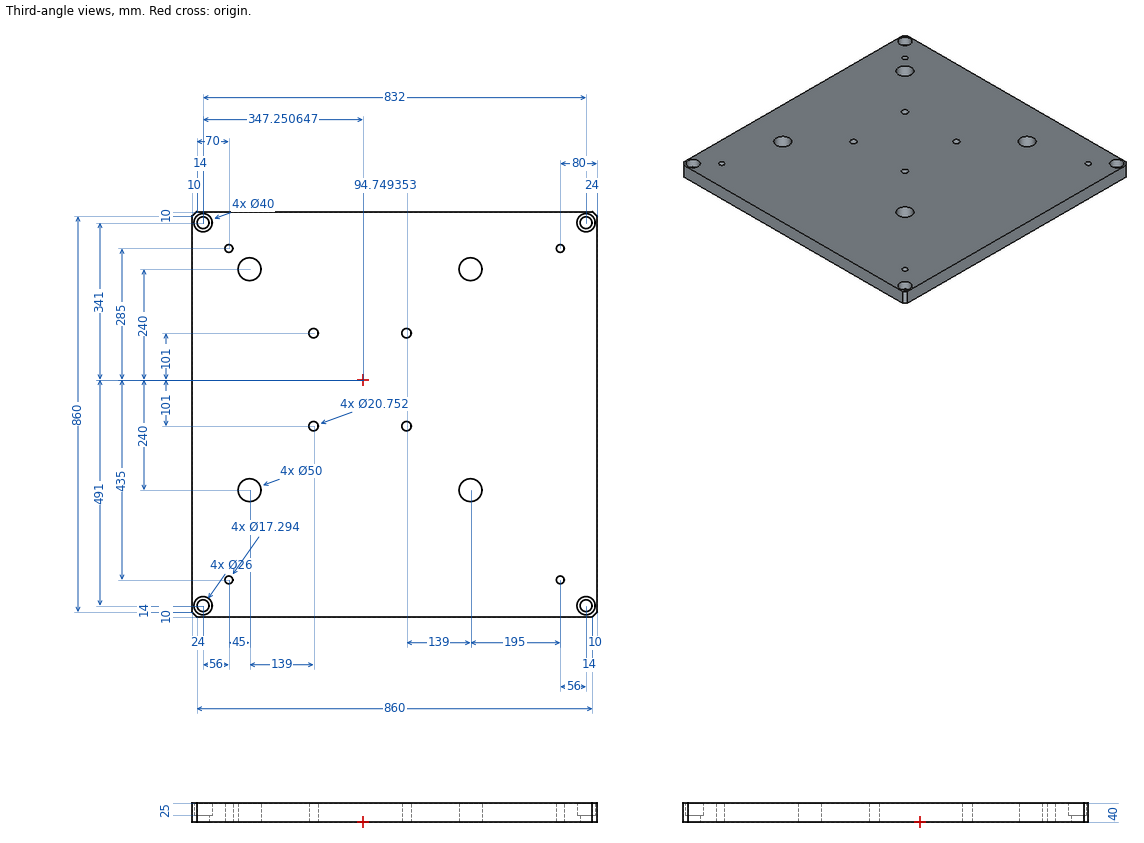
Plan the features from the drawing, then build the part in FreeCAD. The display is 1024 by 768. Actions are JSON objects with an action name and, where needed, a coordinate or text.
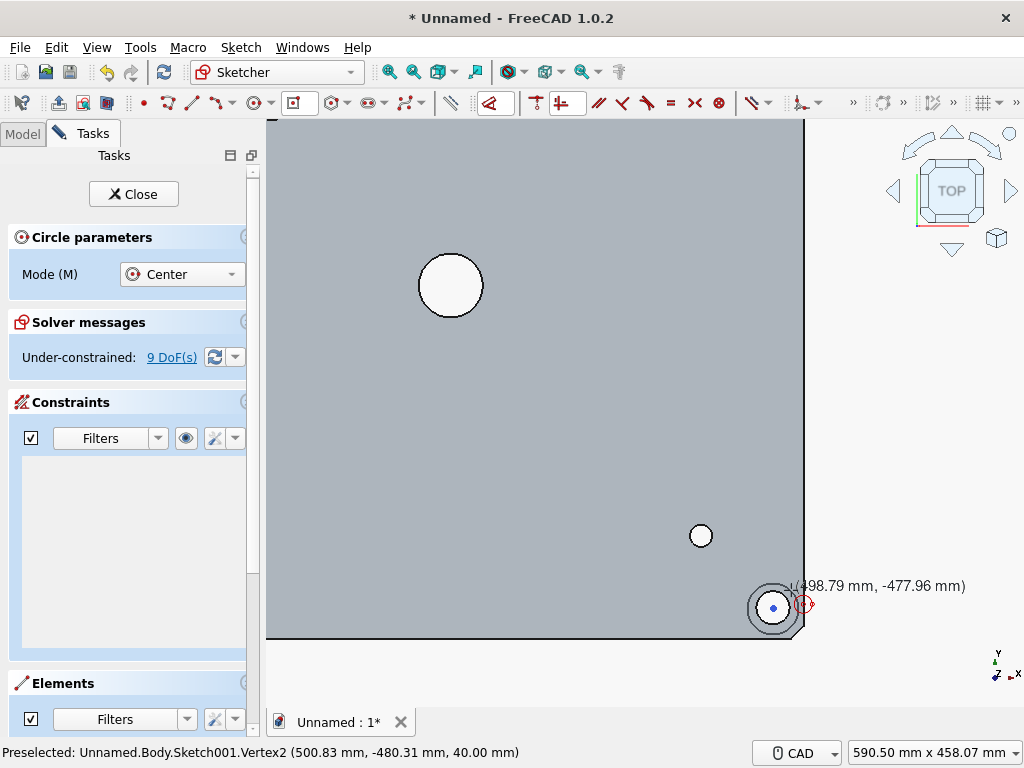
{"action": "scroll", "coordinate": [773, 610], "scroll_direction": "down", "scroll_amount": 5}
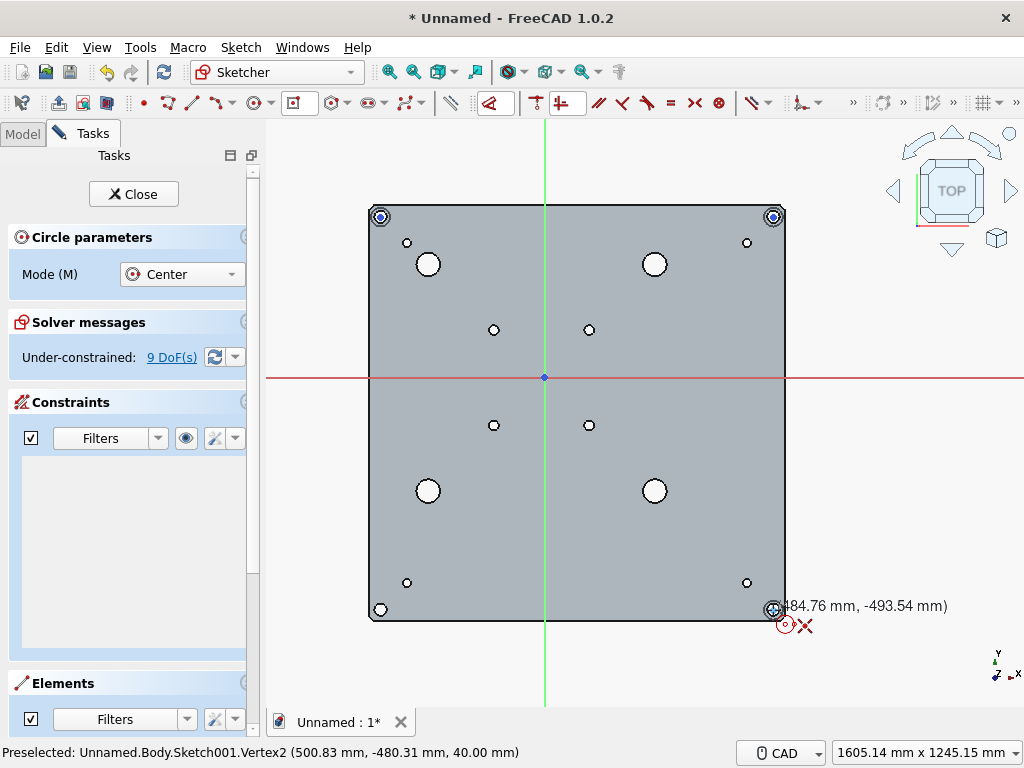
{"action": "scroll", "coordinate": [381, 610], "scroll_direction": "up", "scroll_amount": 5}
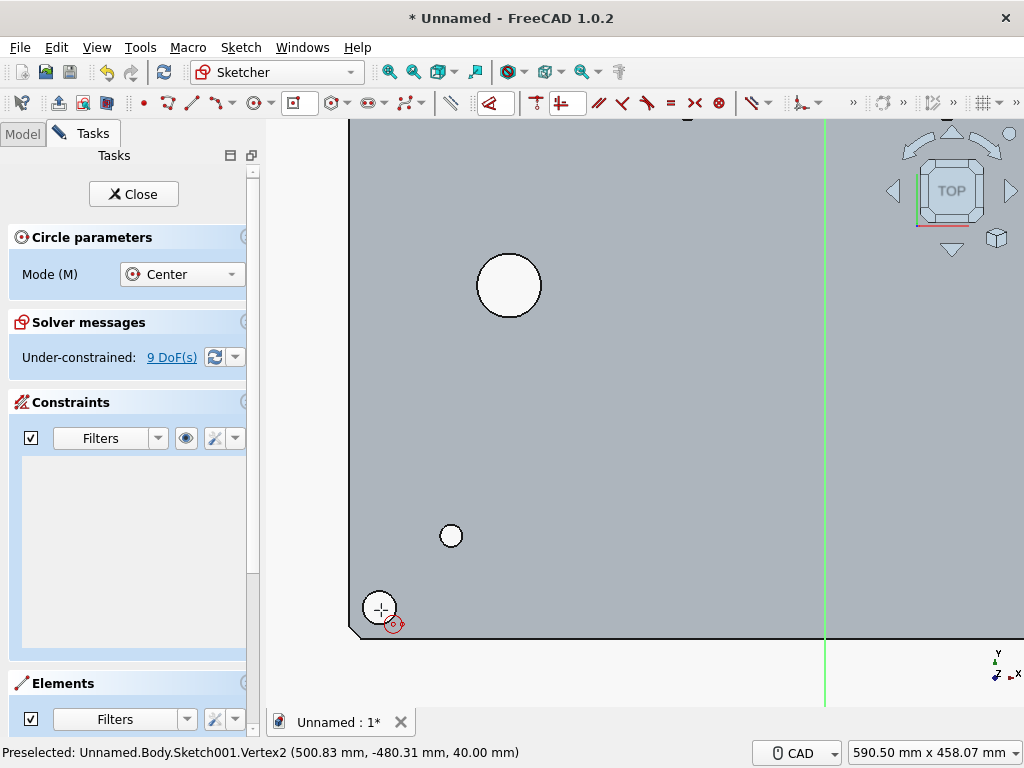
{"action": "left_click", "coordinate": [379, 608]}
{"action": "left_click", "coordinate": [398, 590]}
{"action": "key", "text": "Escape"}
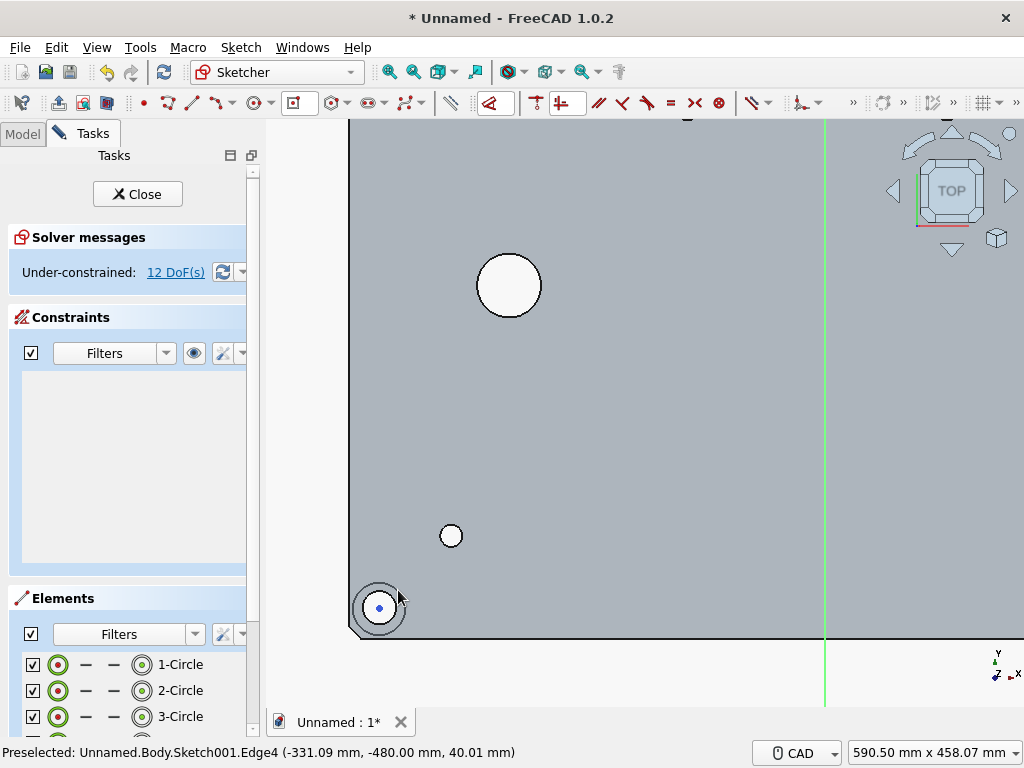
{"action": "scroll", "coordinate": [380, 610], "scroll_direction": "down", "scroll_amount": 5}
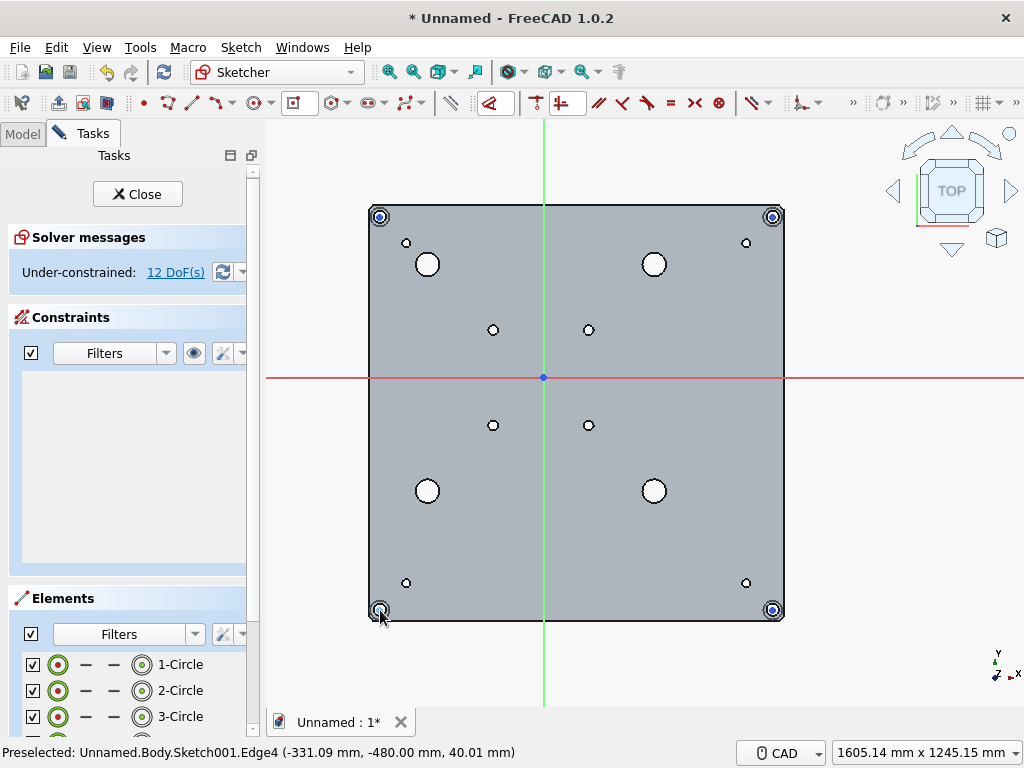
{"action": "scroll", "coordinate": [386, 210], "scroll_direction": "up", "scroll_amount": 2}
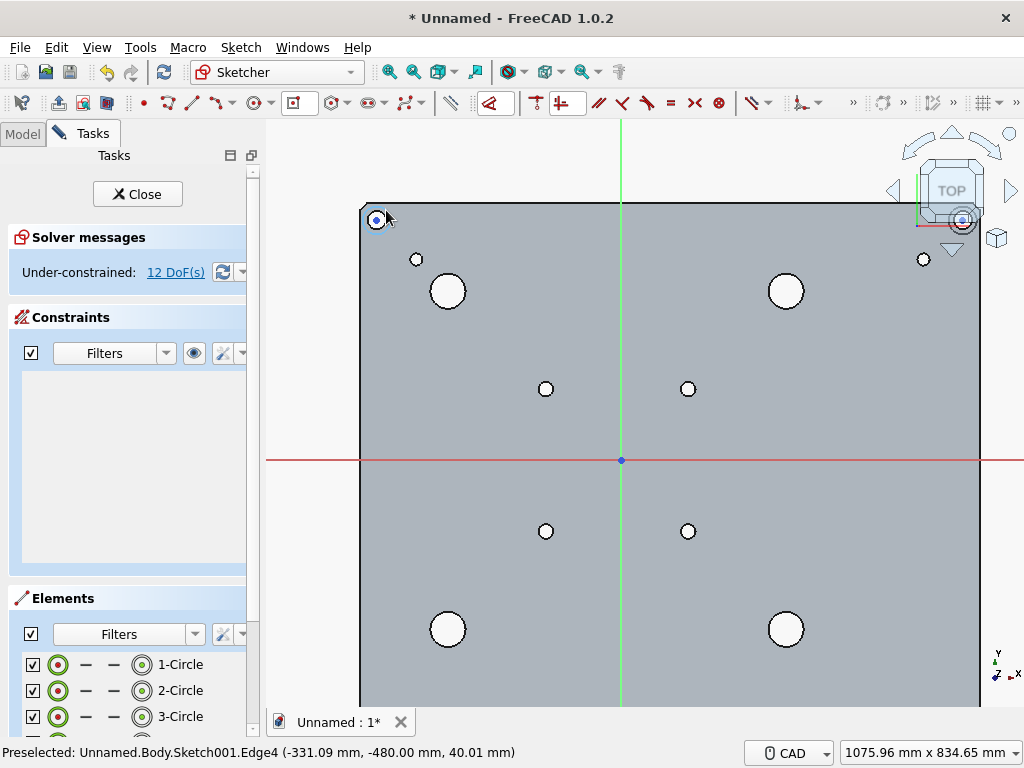
{"action": "left_click", "coordinate": [387, 211]}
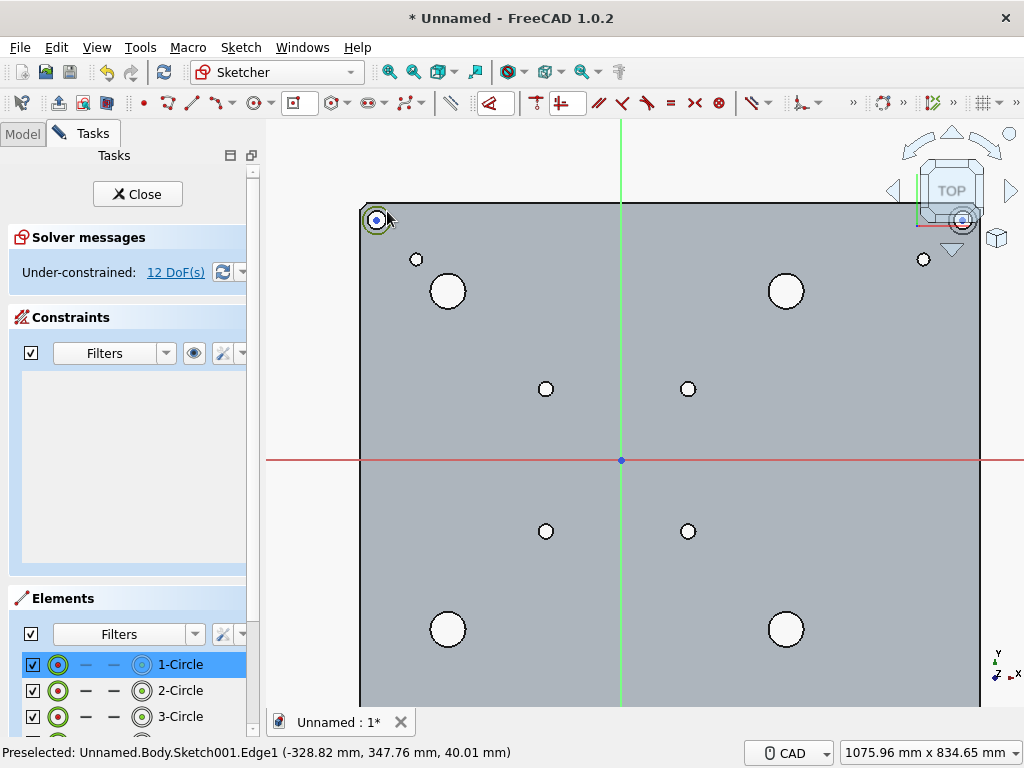
{"action": "scroll", "coordinate": [387, 209], "scroll_direction": "down", "scroll_amount": 2}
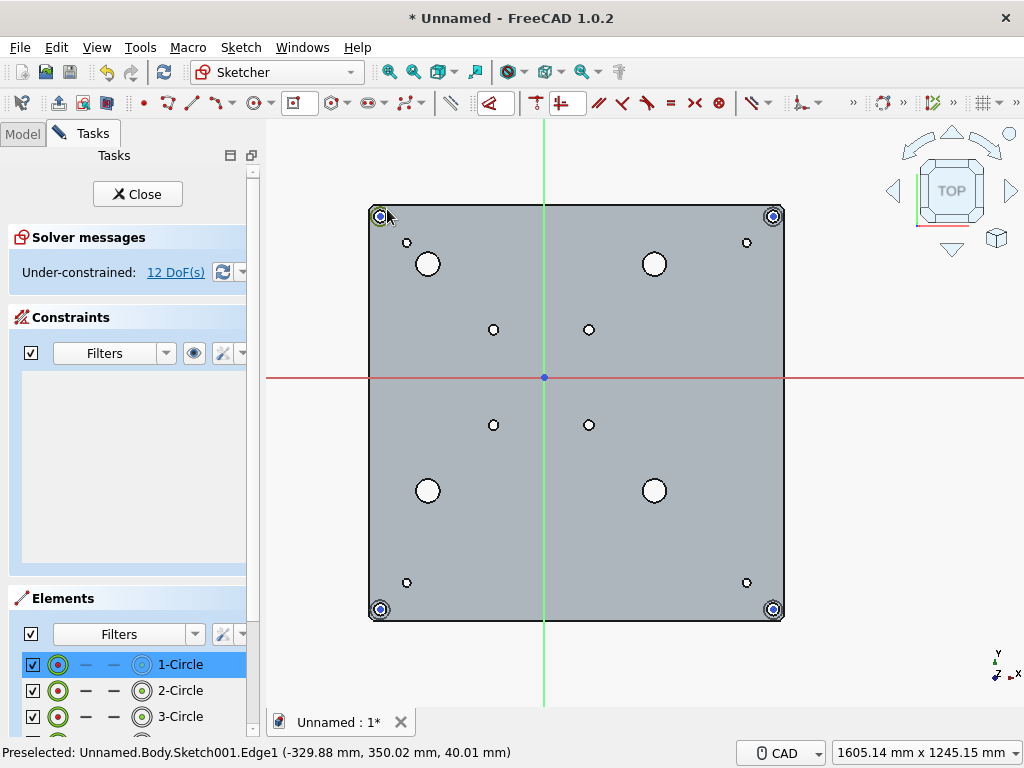
{"action": "scroll", "coordinate": [780, 210], "scroll_direction": "up", "scroll_amount": 2}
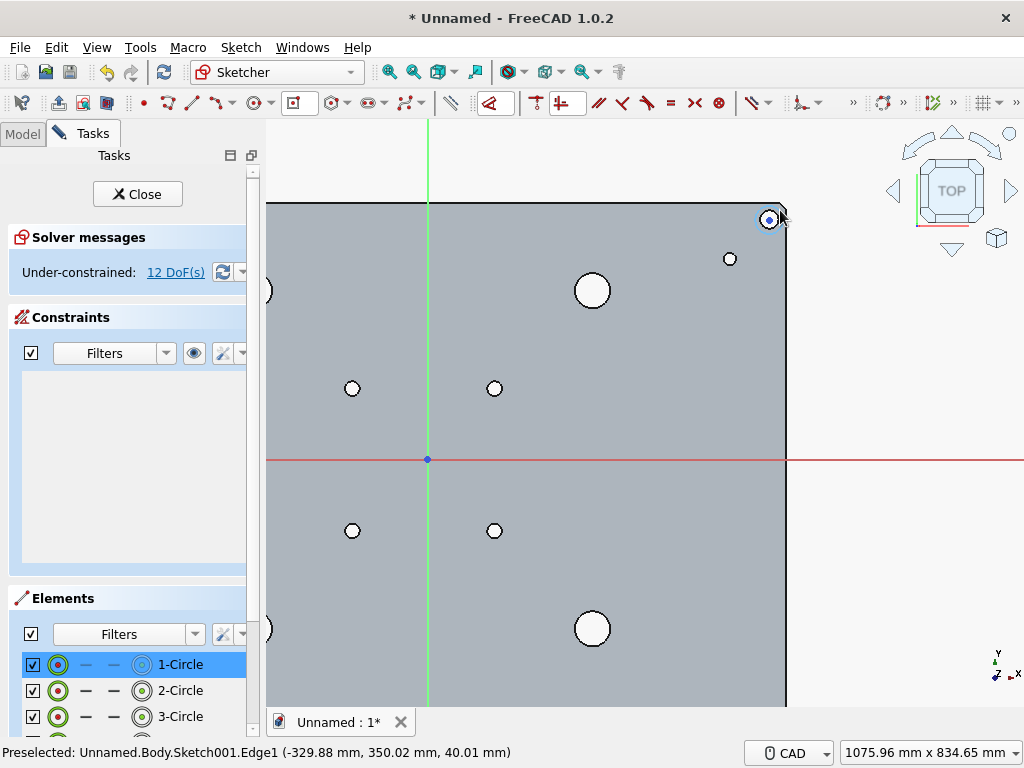
{"action": "left_click", "coordinate": [779, 210]}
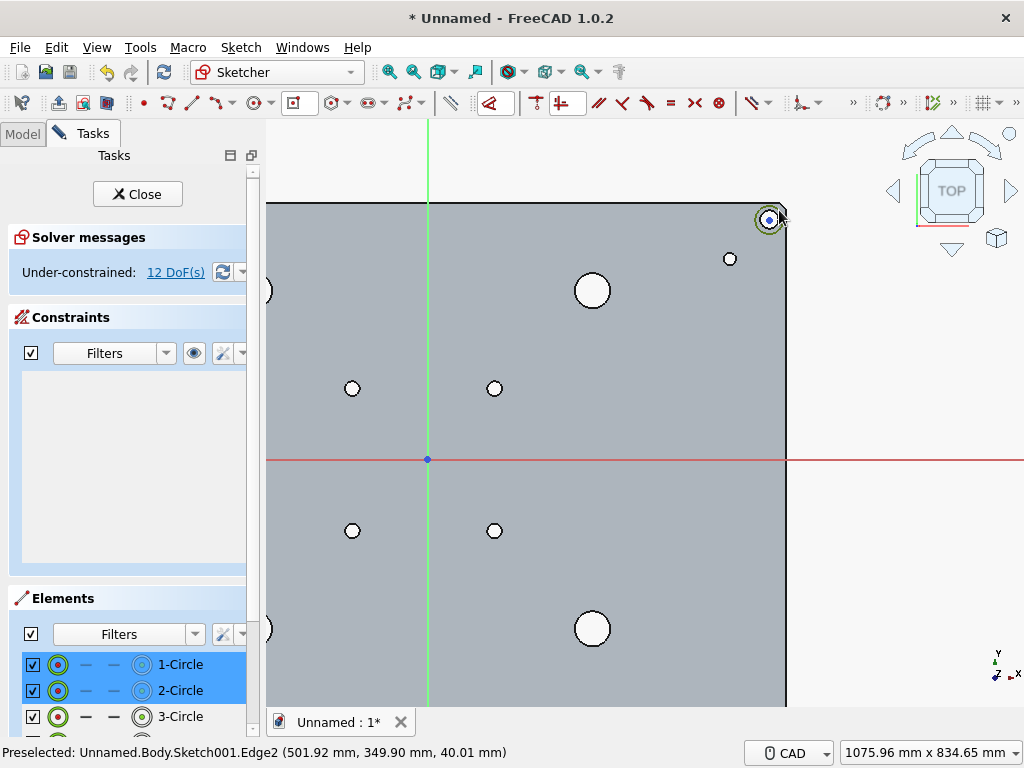
{"action": "scroll", "coordinate": [780, 210], "scroll_direction": "down", "scroll_amount": 2}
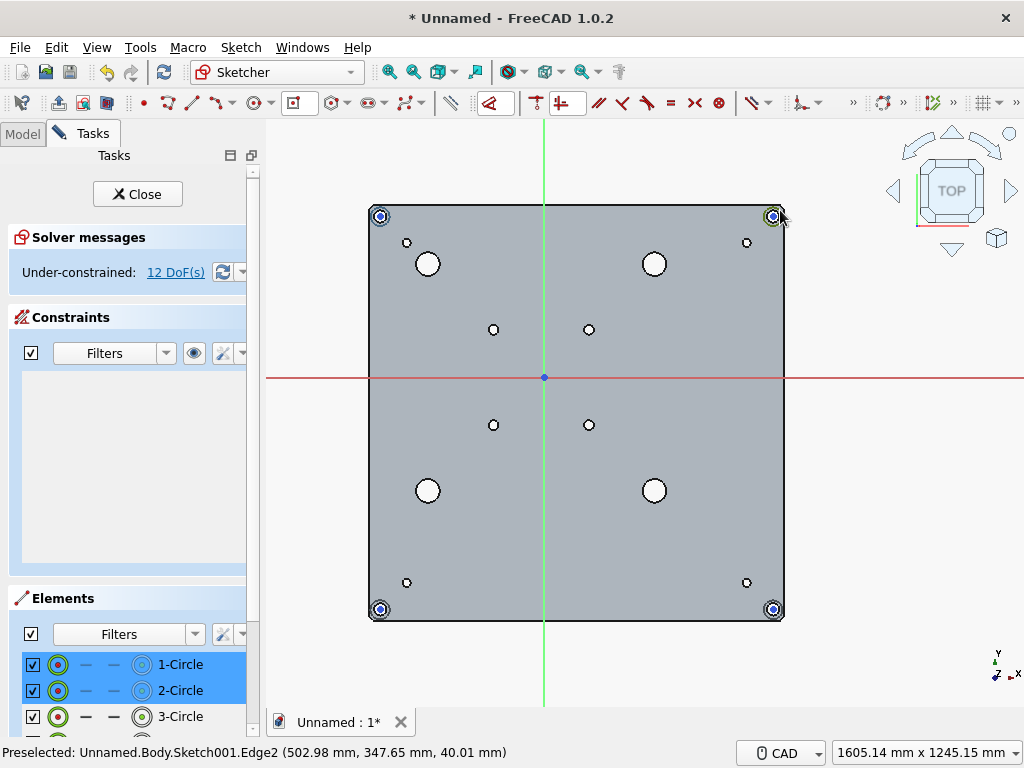
{"action": "scroll", "coordinate": [780, 603], "scroll_direction": "up", "scroll_amount": 2}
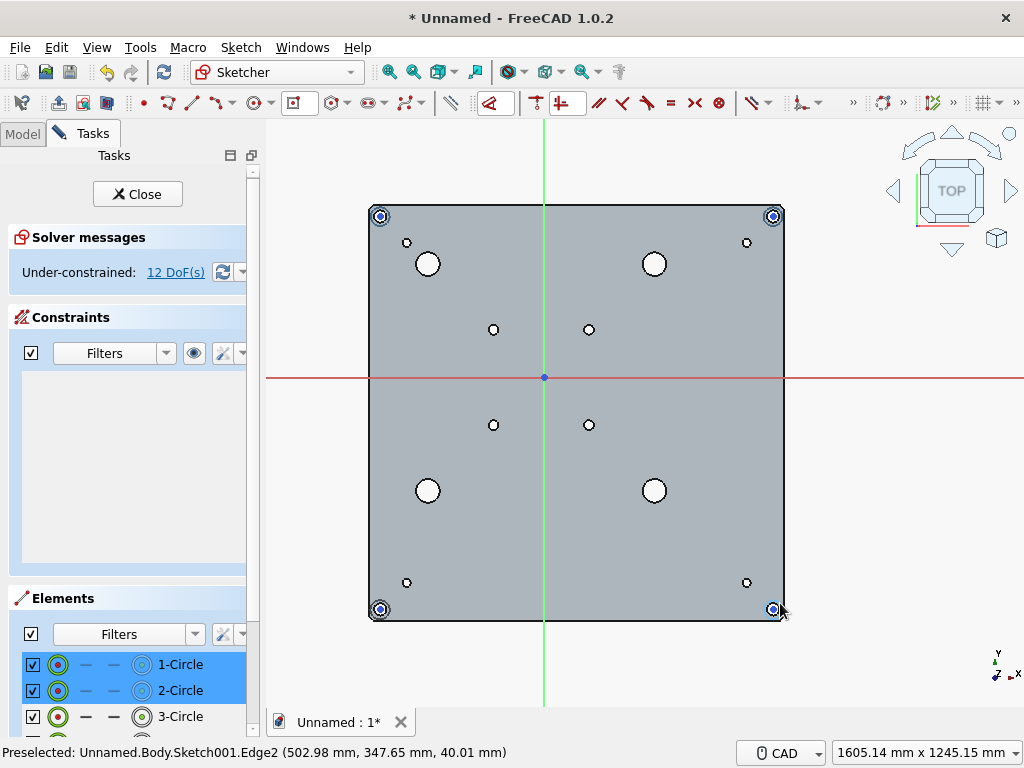
{"action": "left_click", "coordinate": [779, 603]}